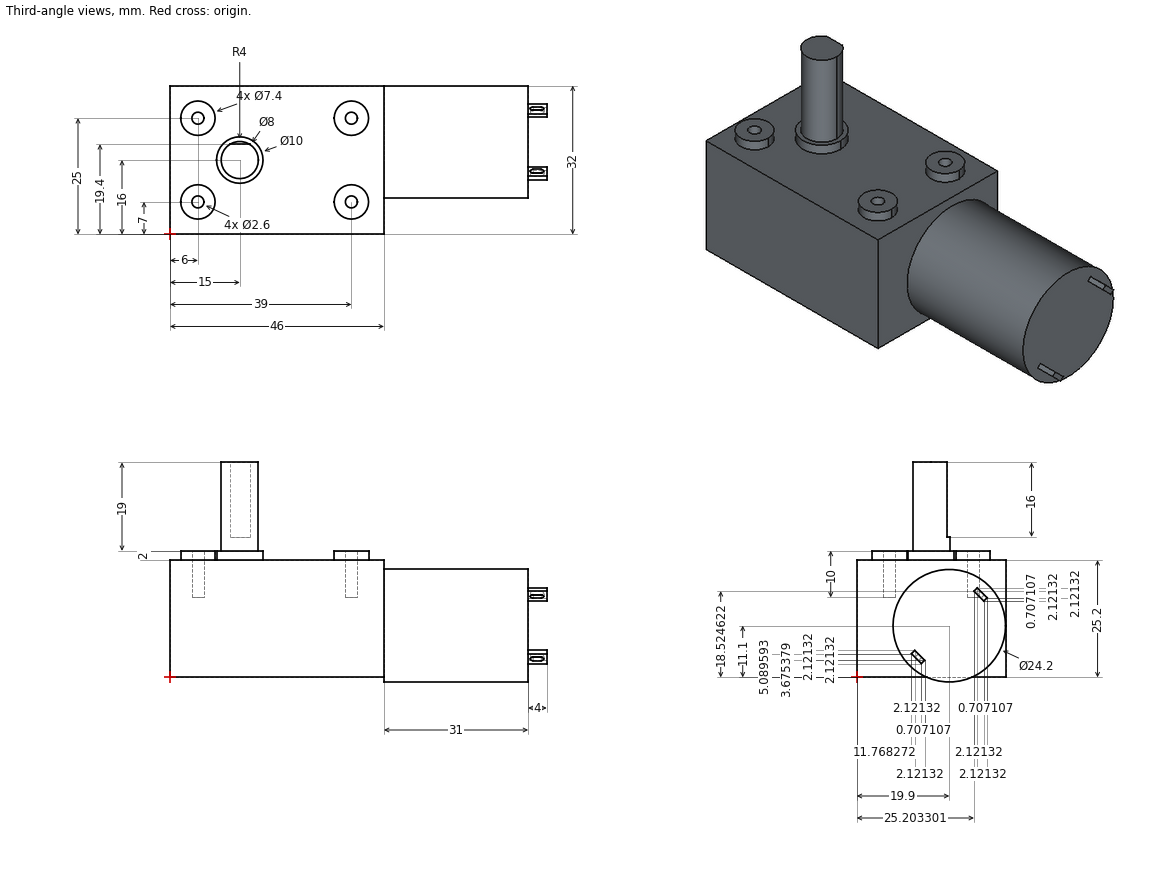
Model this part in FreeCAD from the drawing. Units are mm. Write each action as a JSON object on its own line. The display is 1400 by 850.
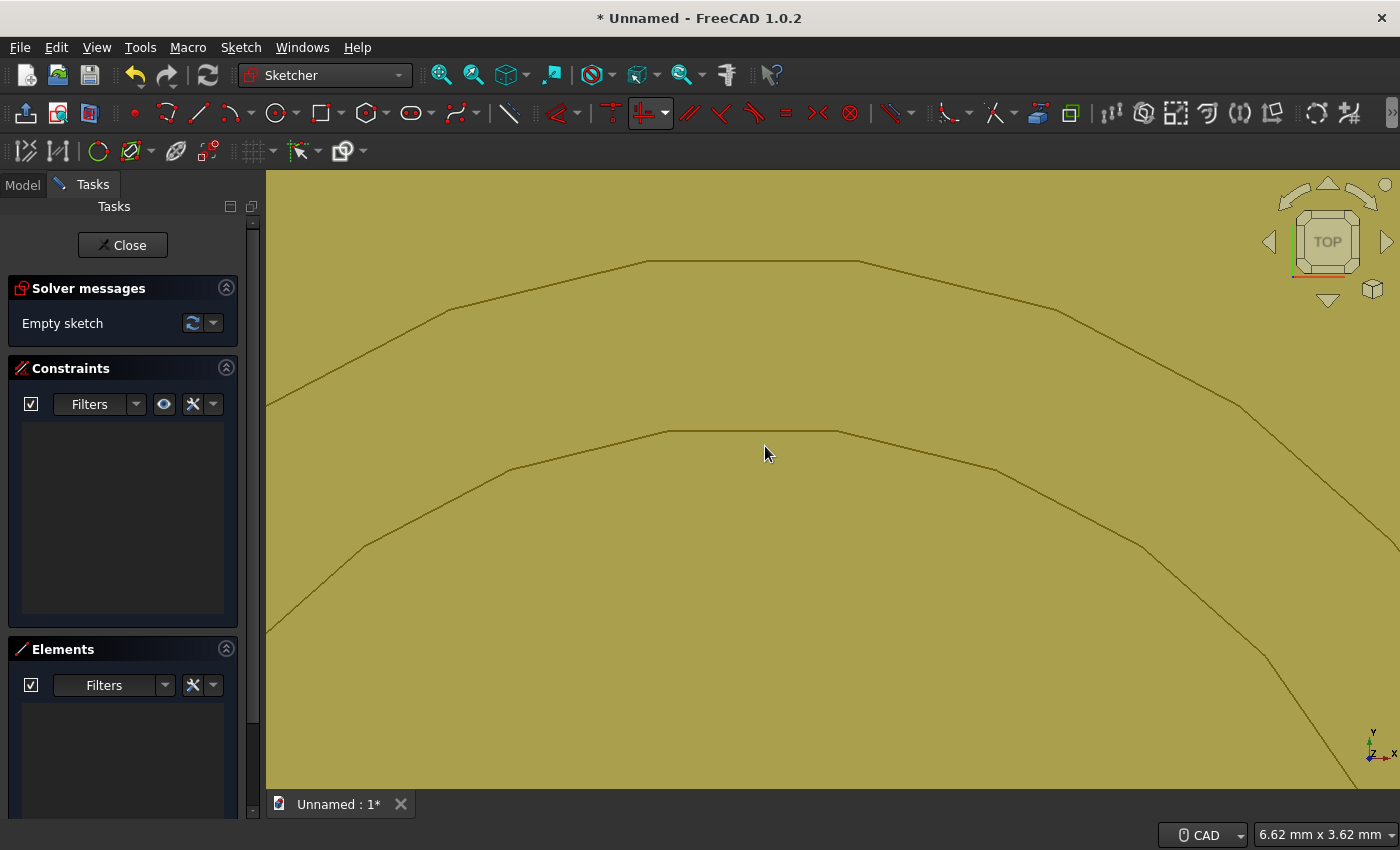
{"action": "key", "text": "g l"}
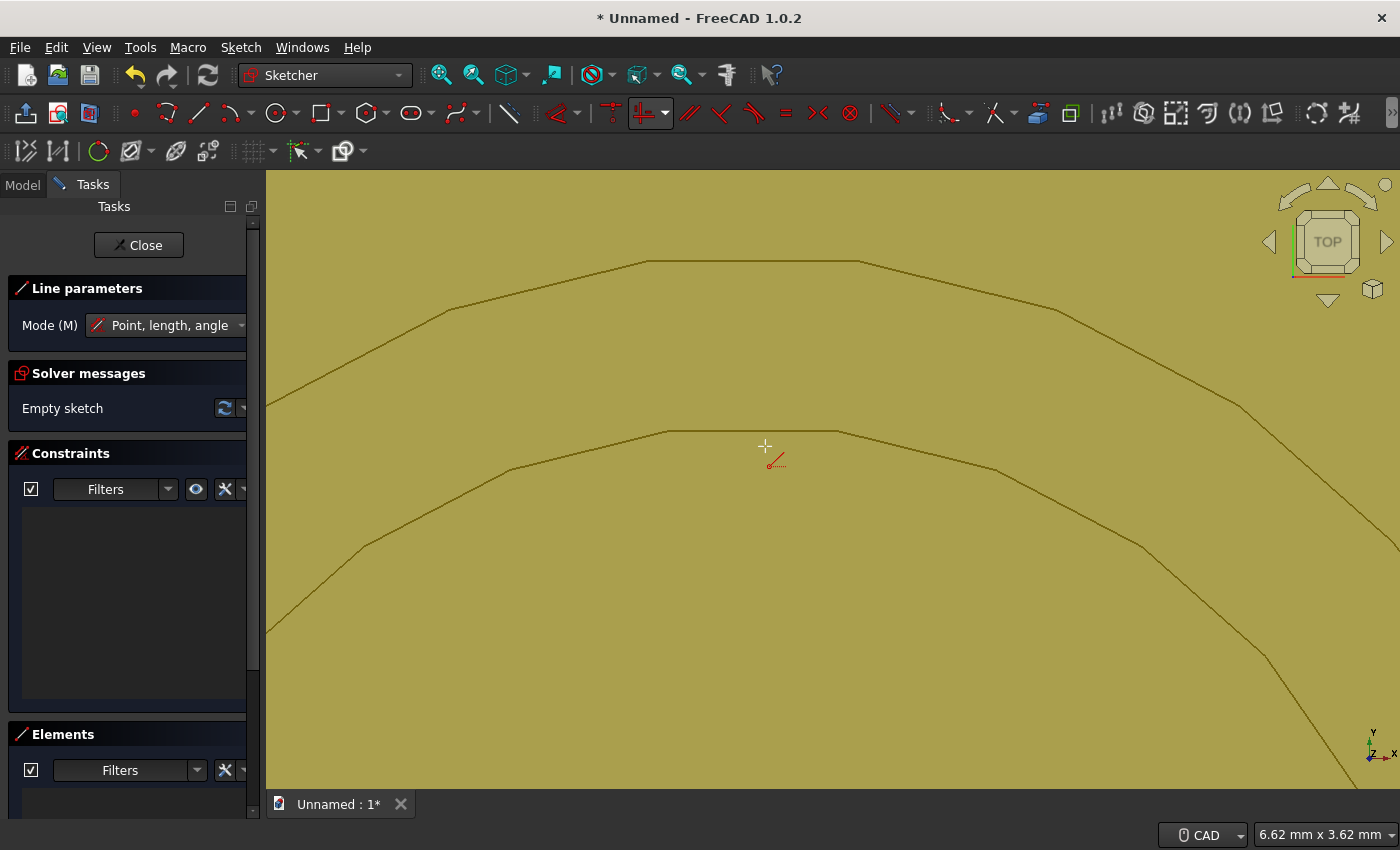
{"action": "left_click", "coordinate": [392, 528]}
{"action": "left_click", "coordinate": [1114, 528]}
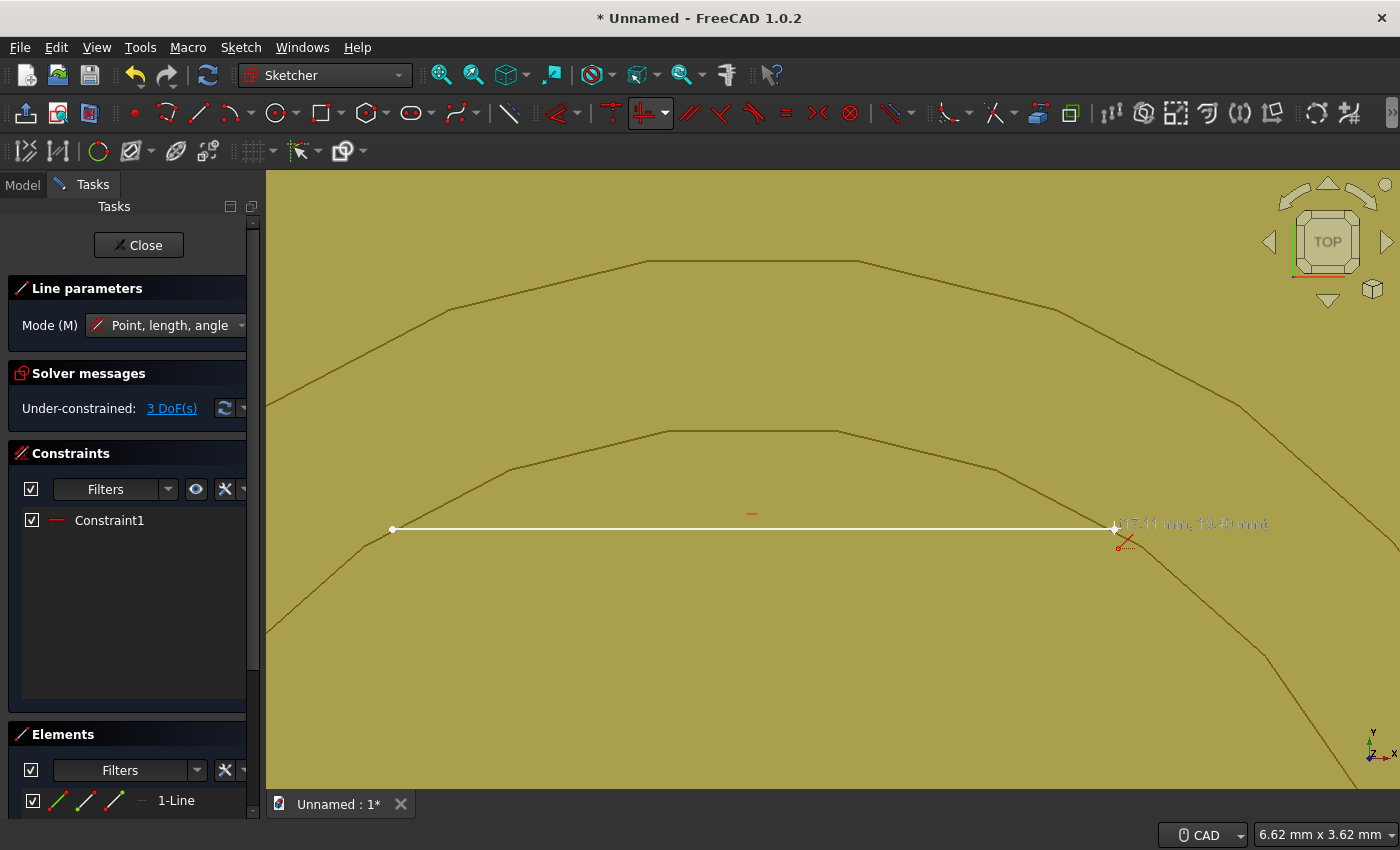
{"action": "left_click", "coordinate": [254, 114]}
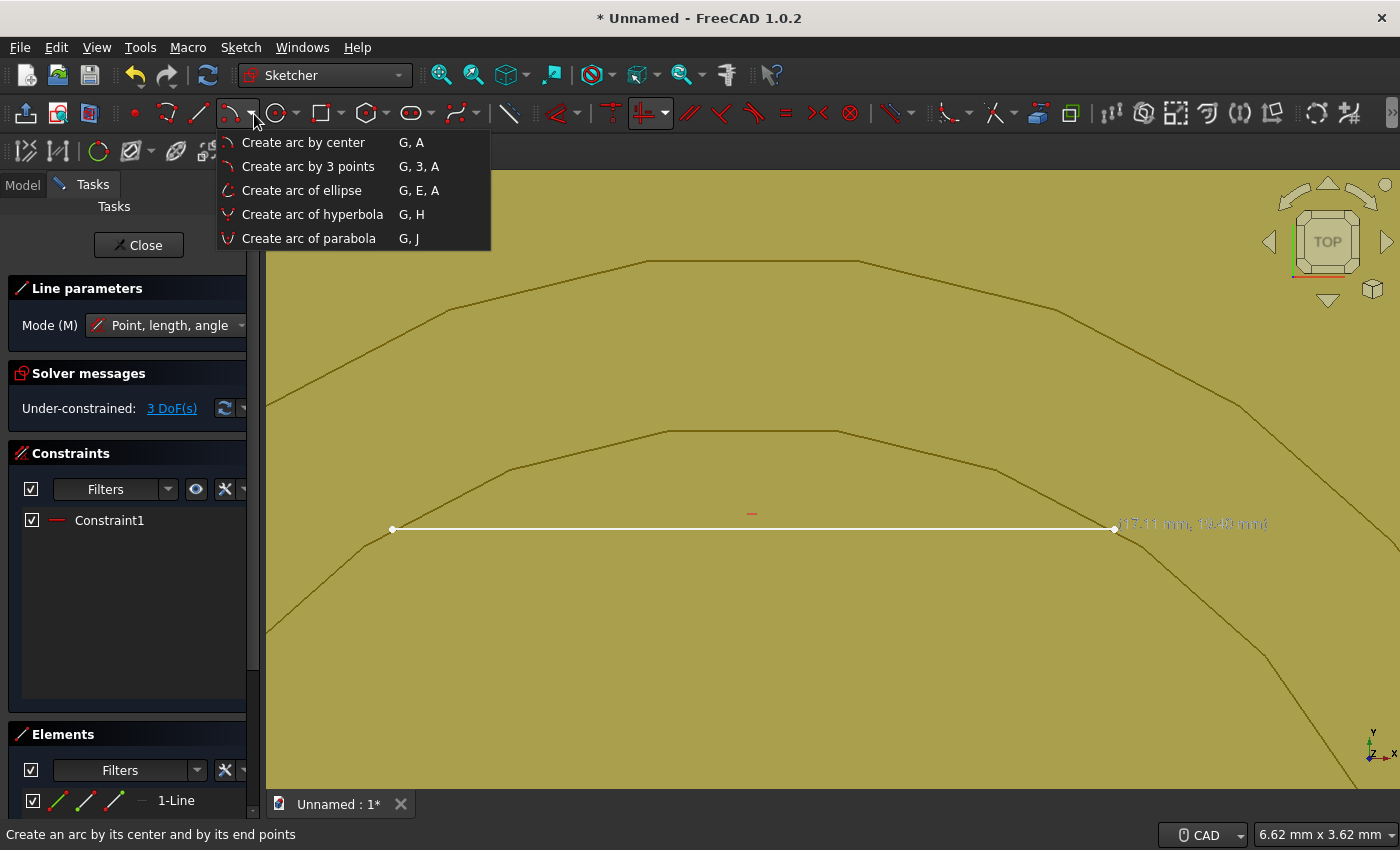
{"action": "left_click", "coordinate": [354, 166]}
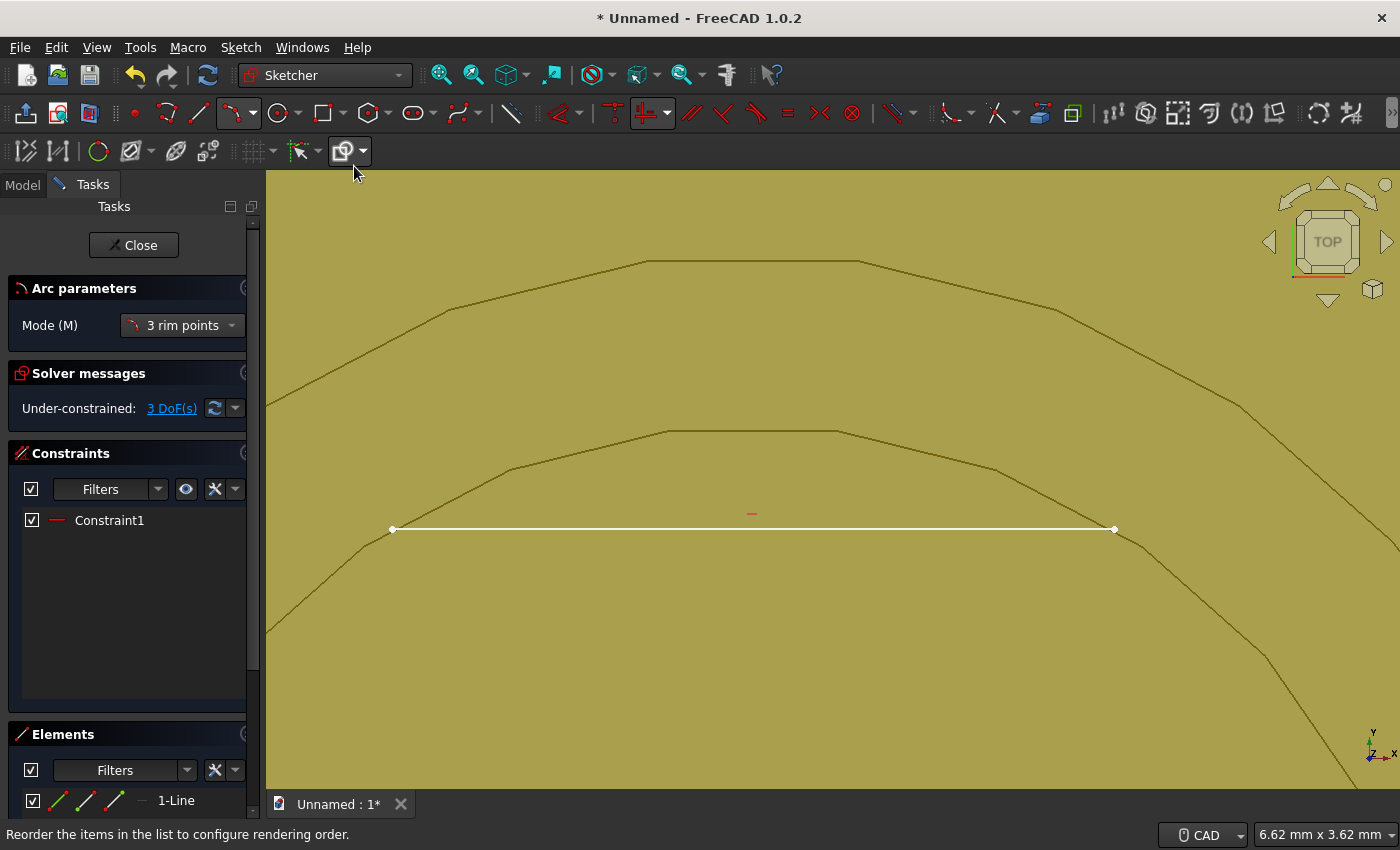
{"action": "left_click", "coordinate": [1114, 529]}
{"action": "left_click", "coordinate": [392, 529]}
{"action": "left_click", "coordinate": [753, 426]}
{"action": "key", "text": "Escape"}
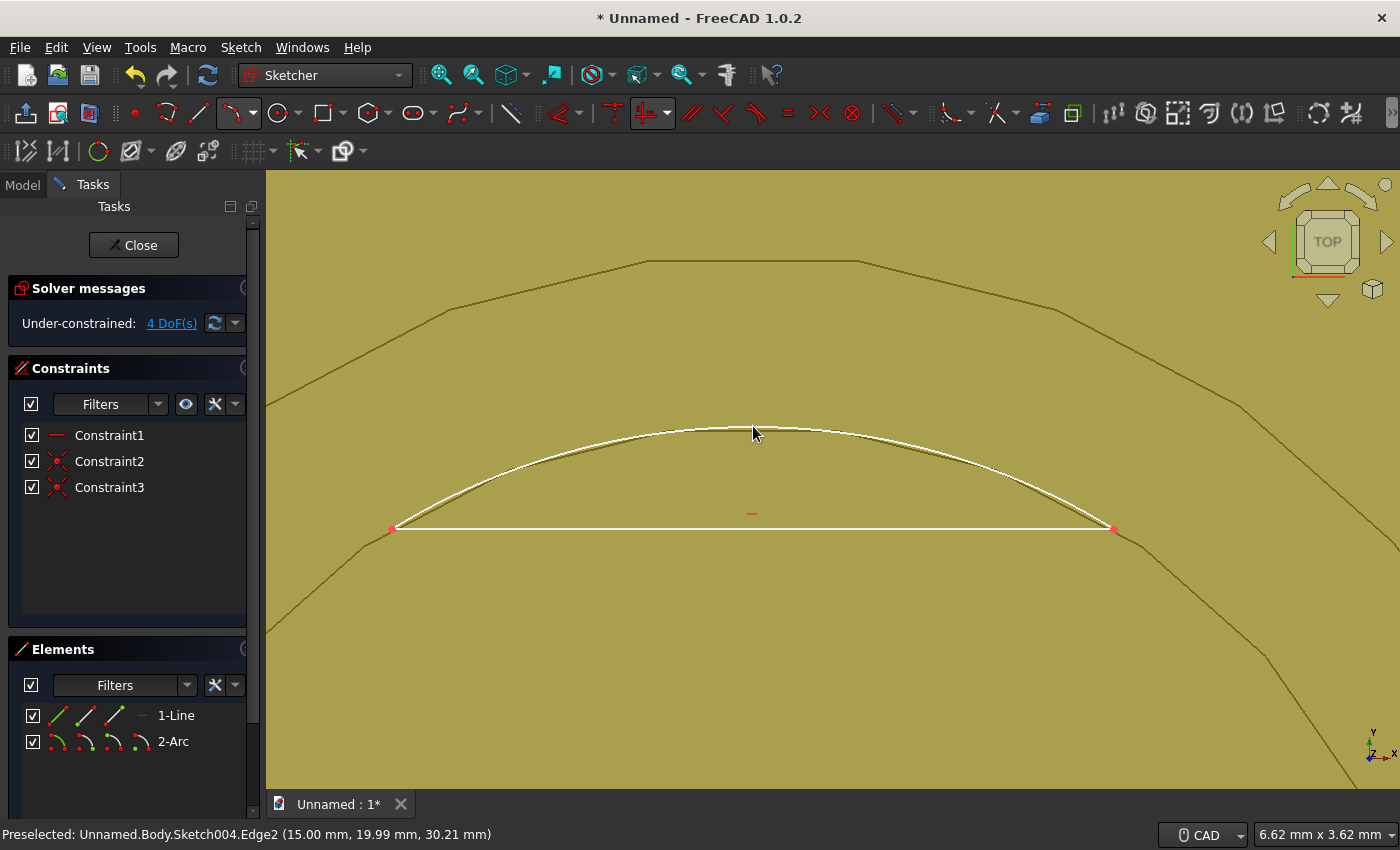
{"action": "left_click", "coordinate": [558, 114]}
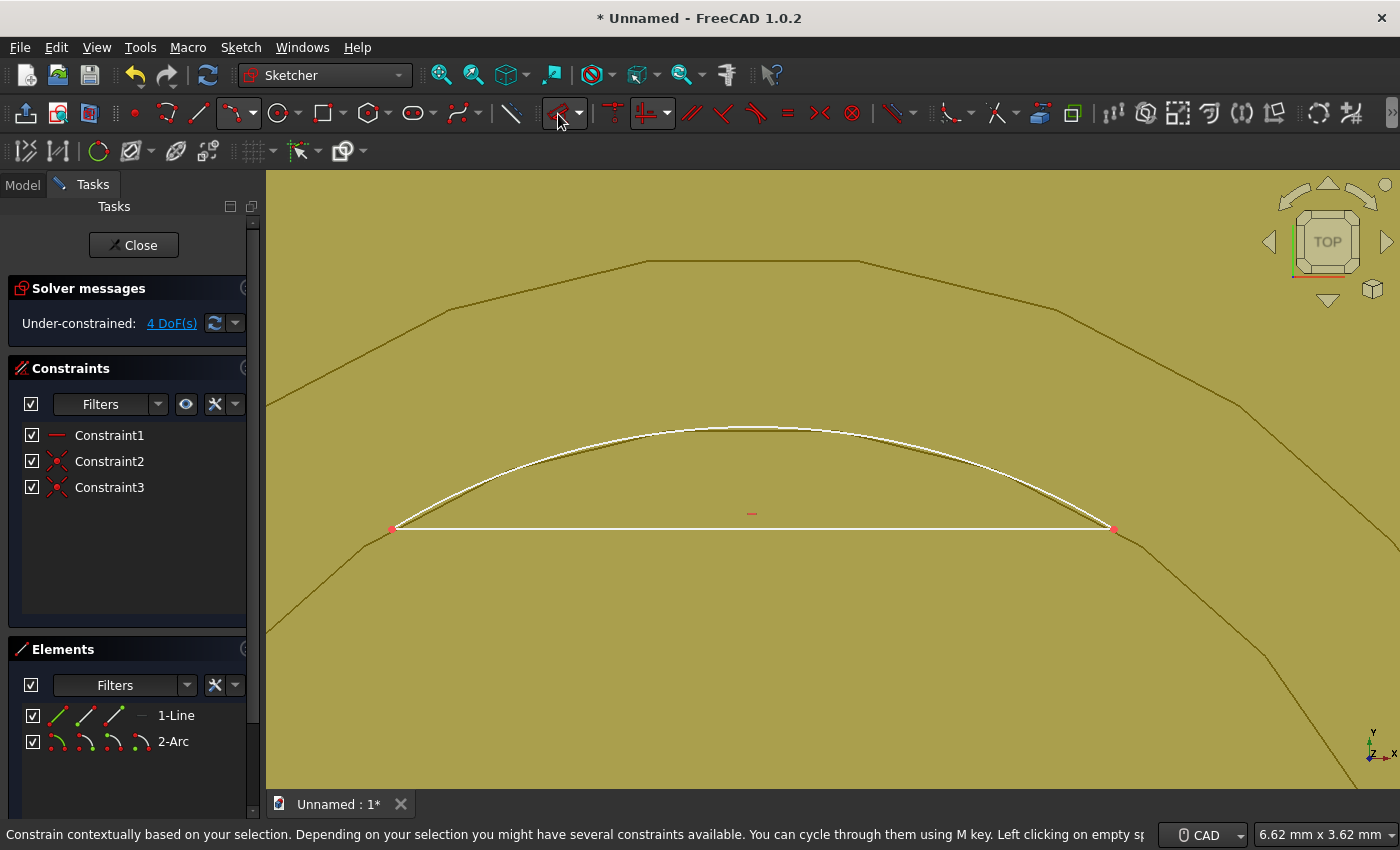
{"action": "left_click", "coordinate": [904, 444]}
{"action": "left_click", "coordinate": [911, 413]}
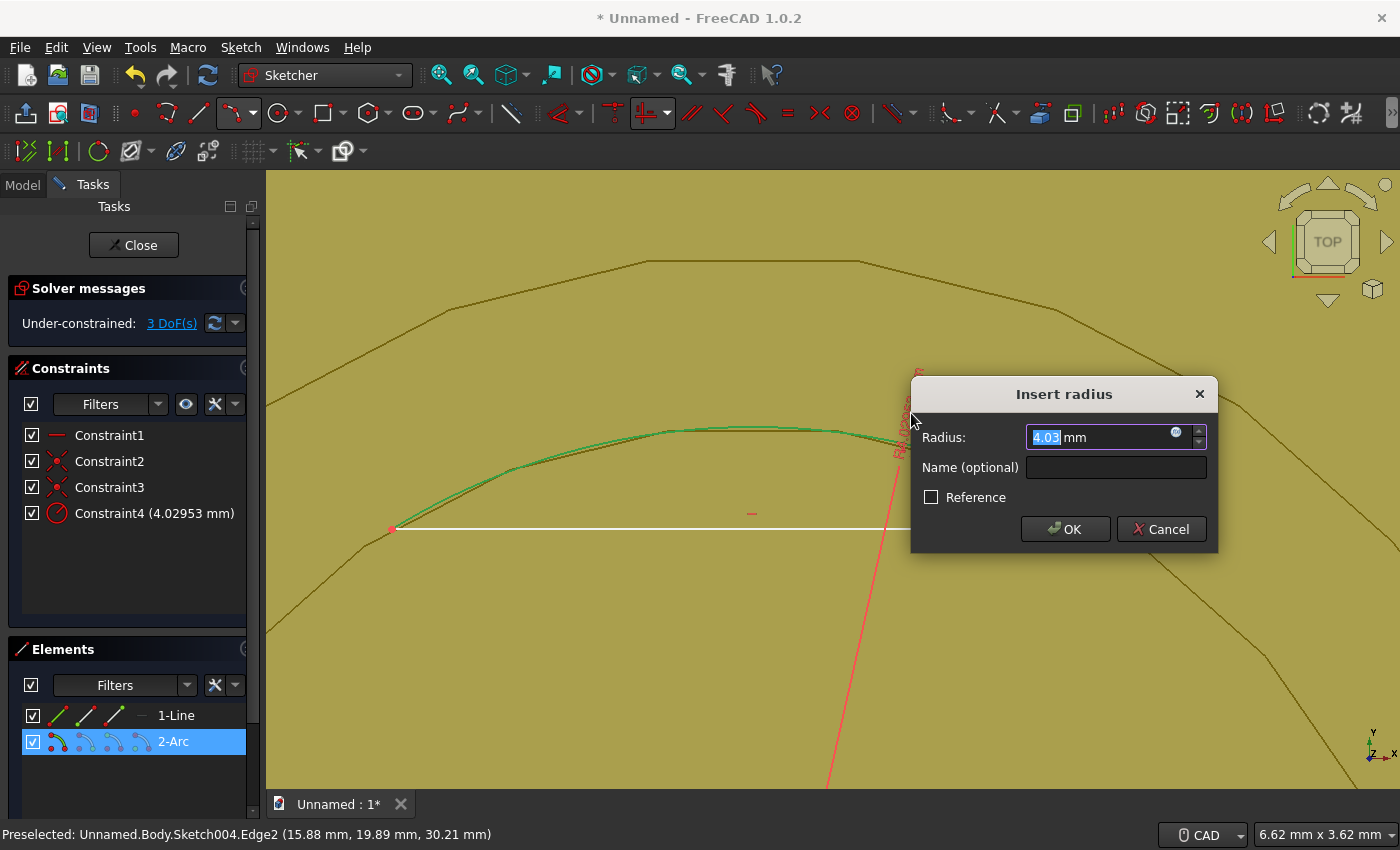
{"action": "type", "text": "4"}
{"action": "key", "text": "Return"}